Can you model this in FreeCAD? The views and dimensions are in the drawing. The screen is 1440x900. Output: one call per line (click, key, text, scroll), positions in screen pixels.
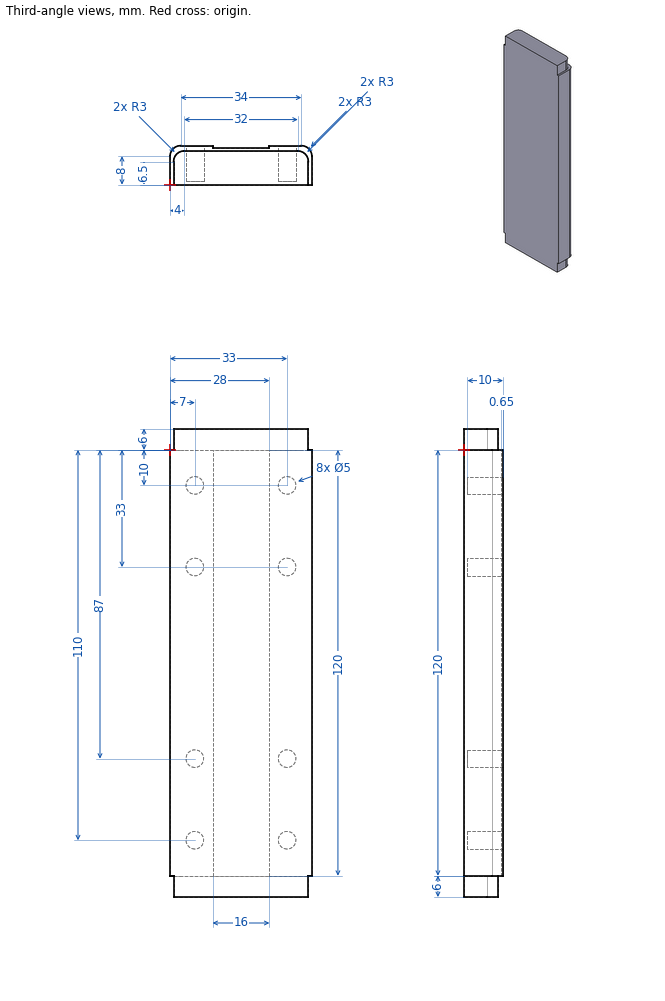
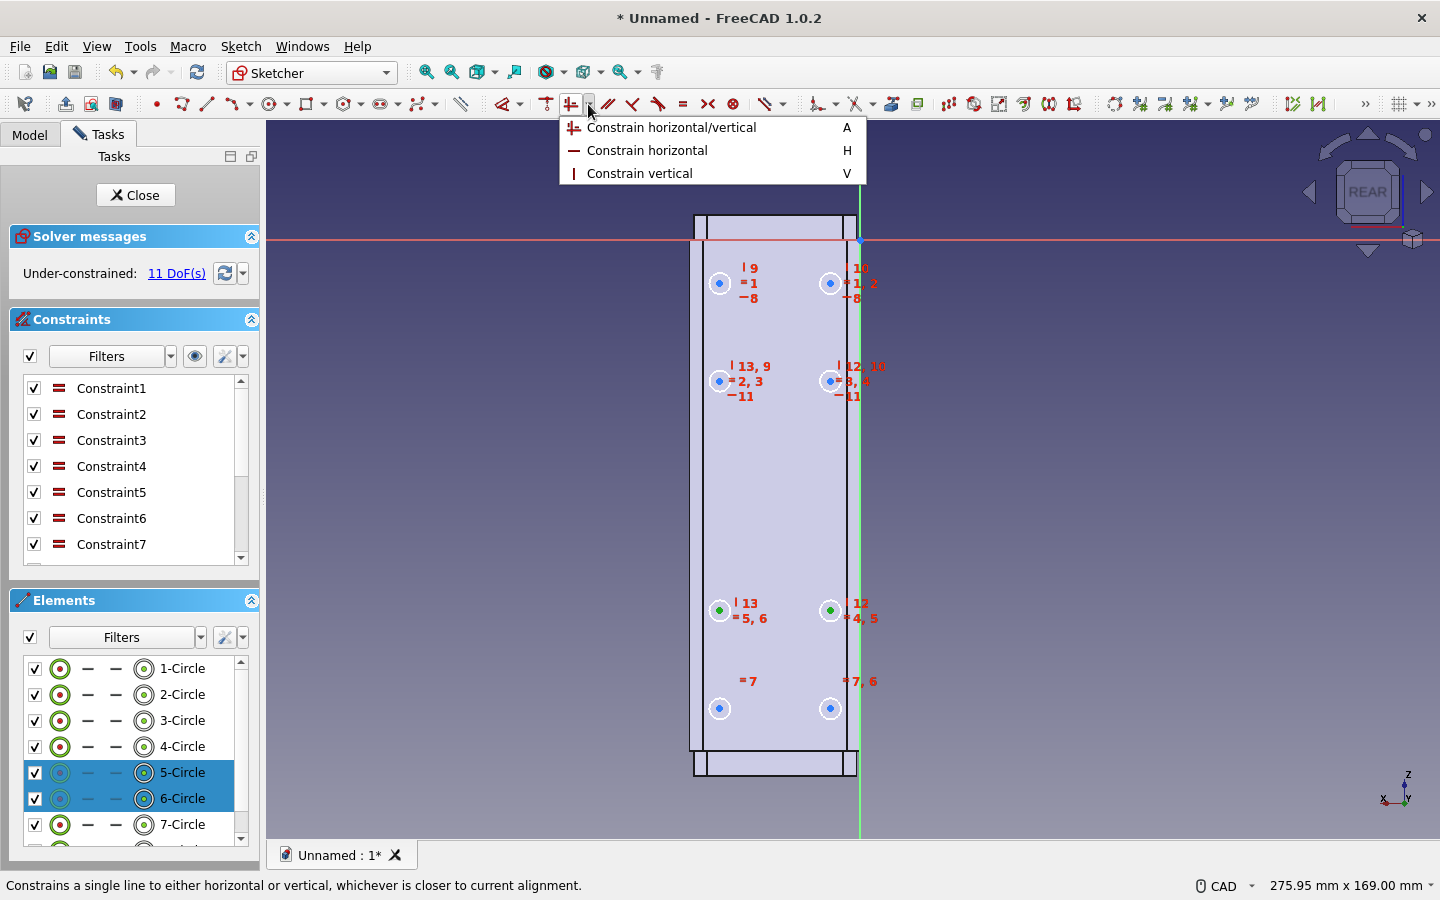
click(713, 150)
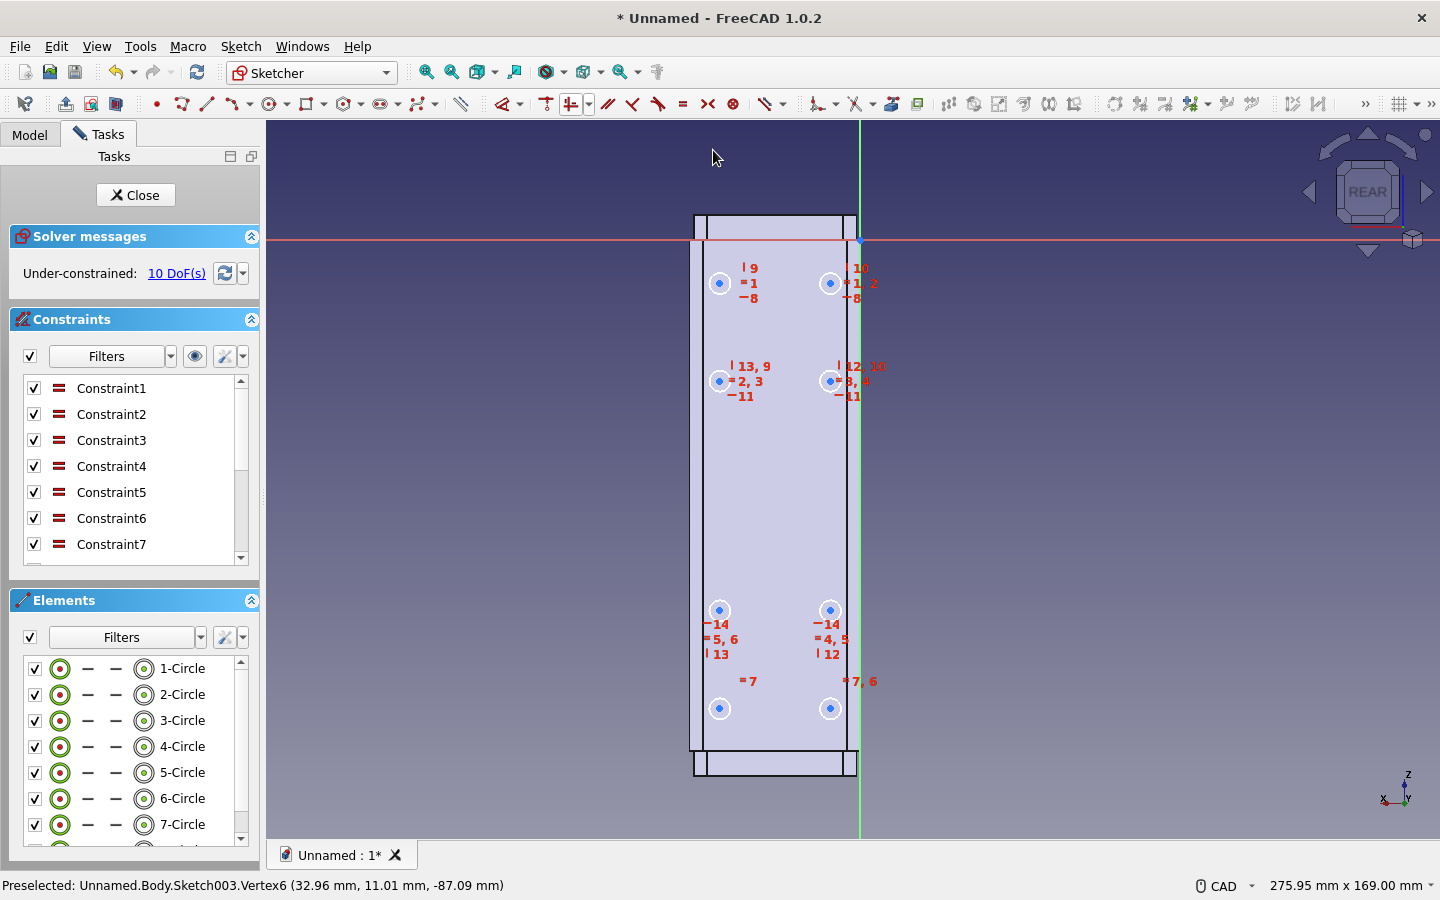
click(831, 611)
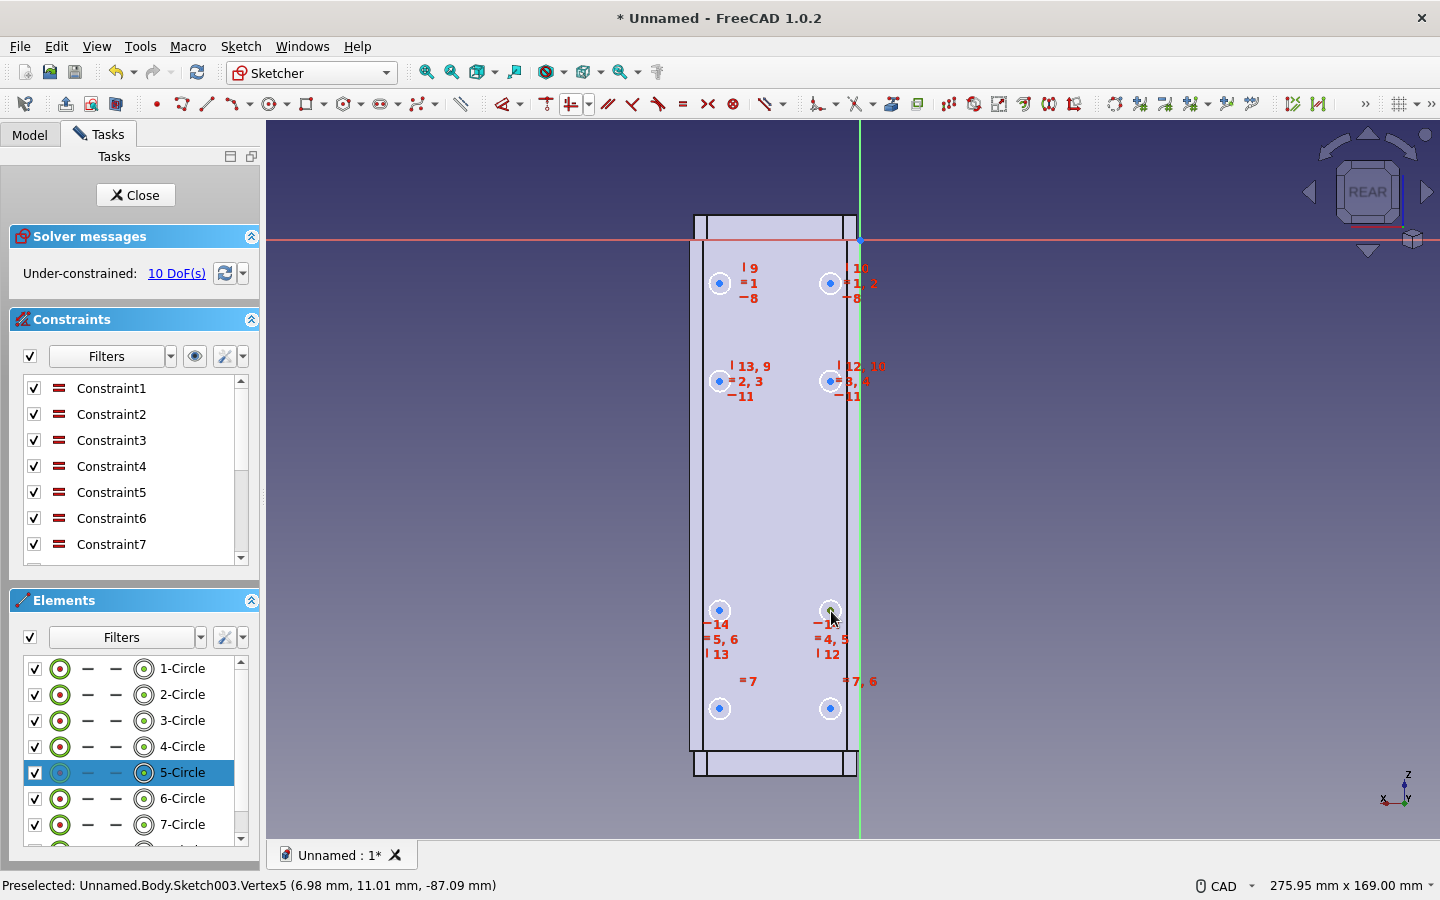
click(830, 709)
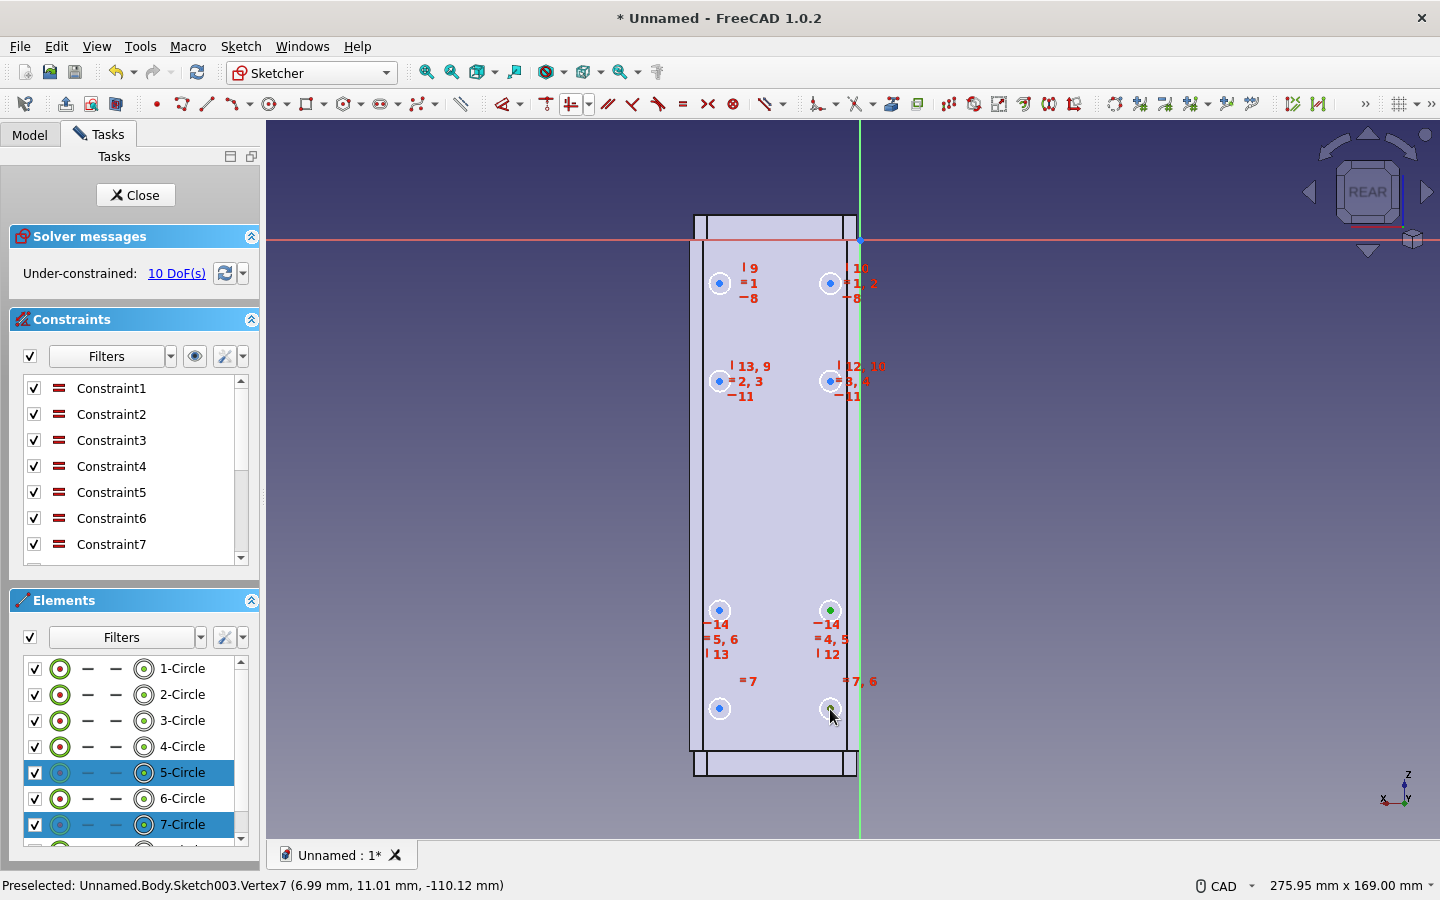
key(v)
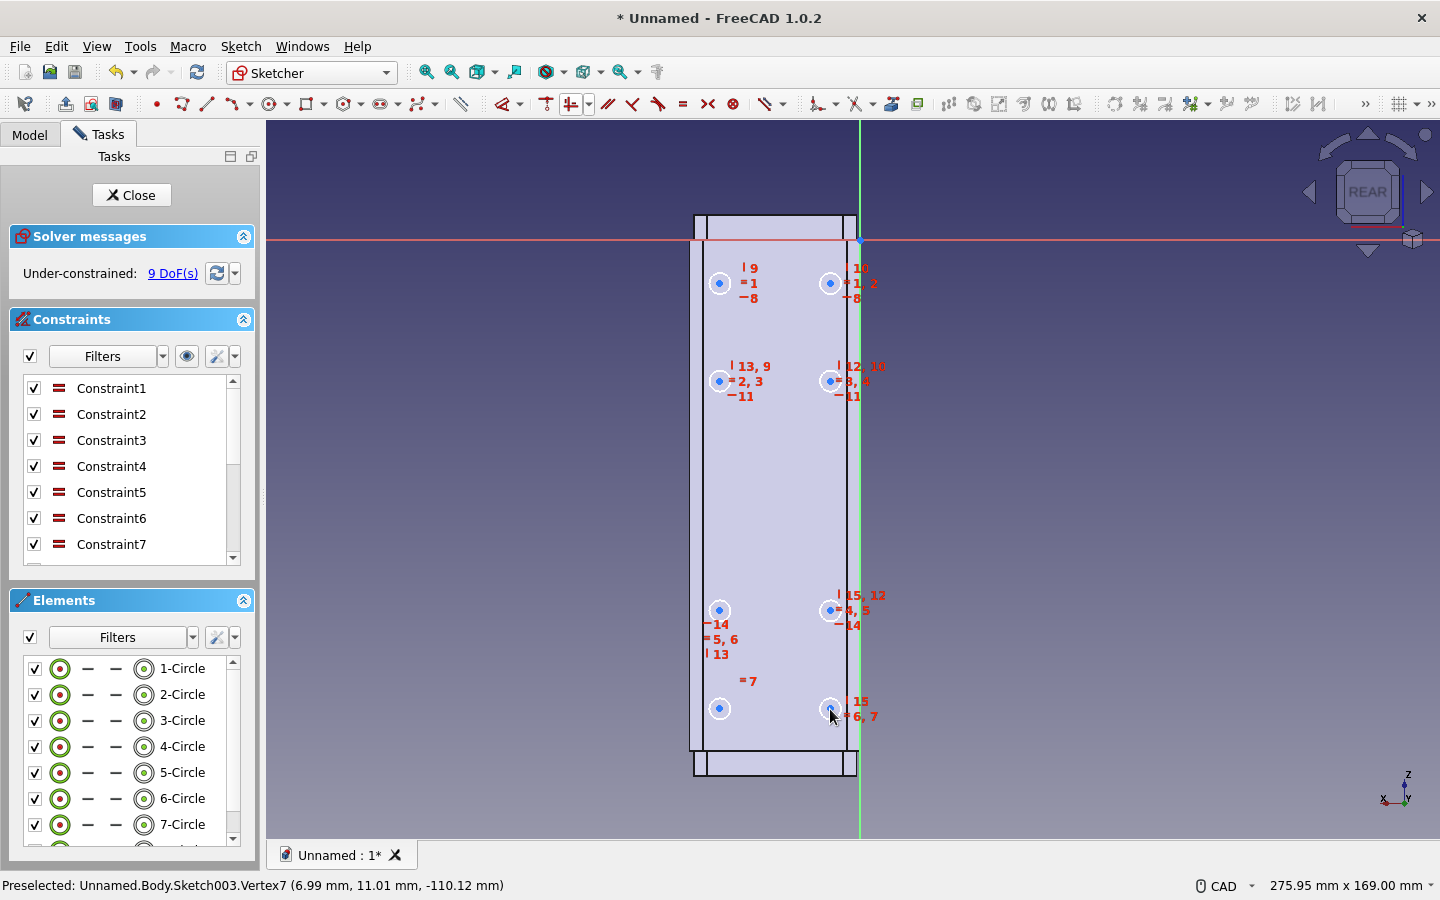
click(720, 611)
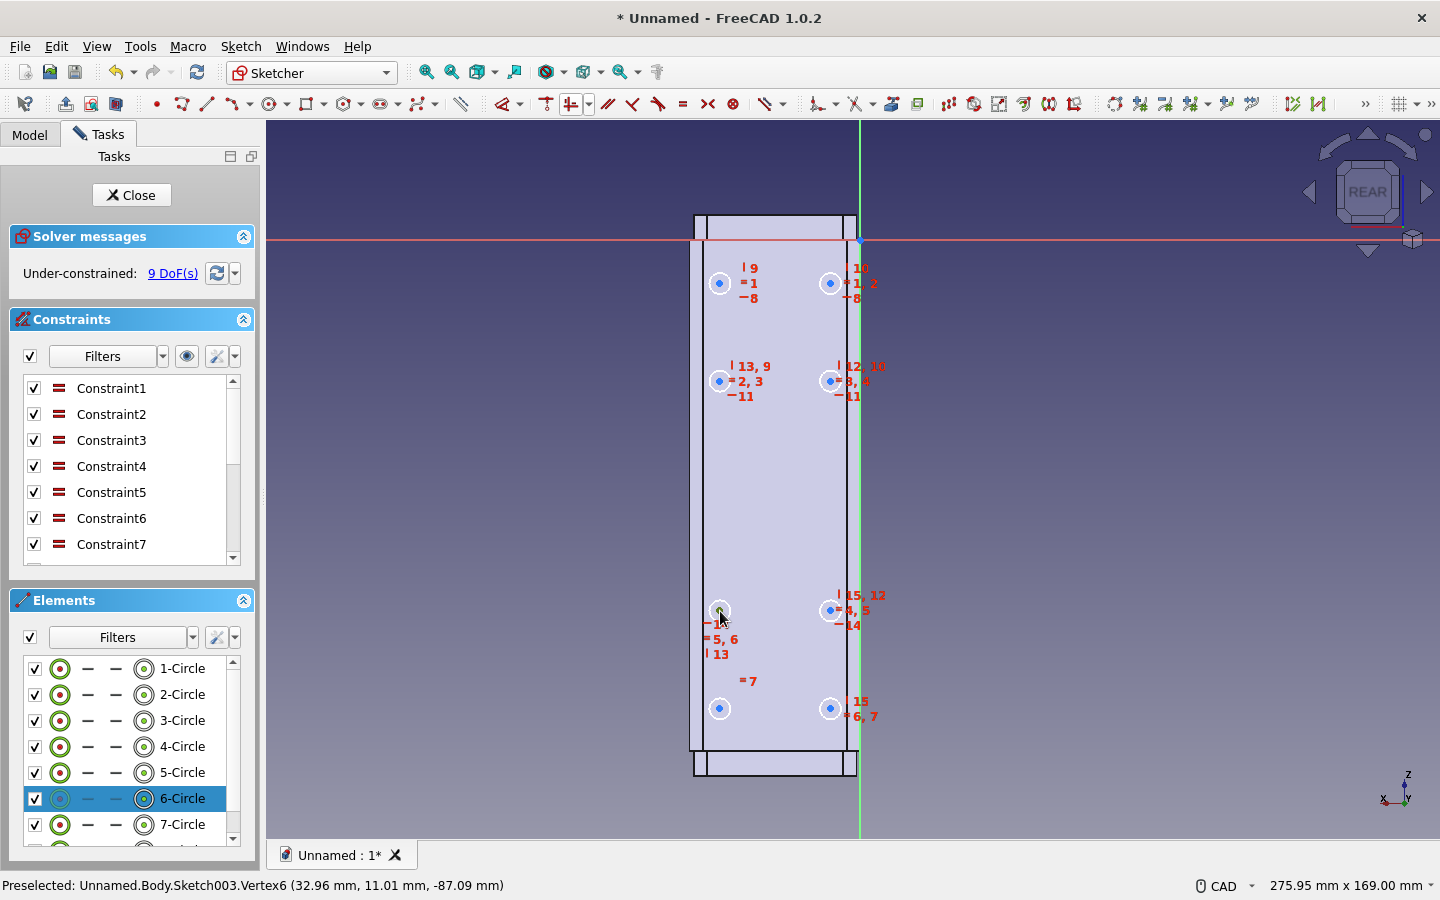
click(720, 709)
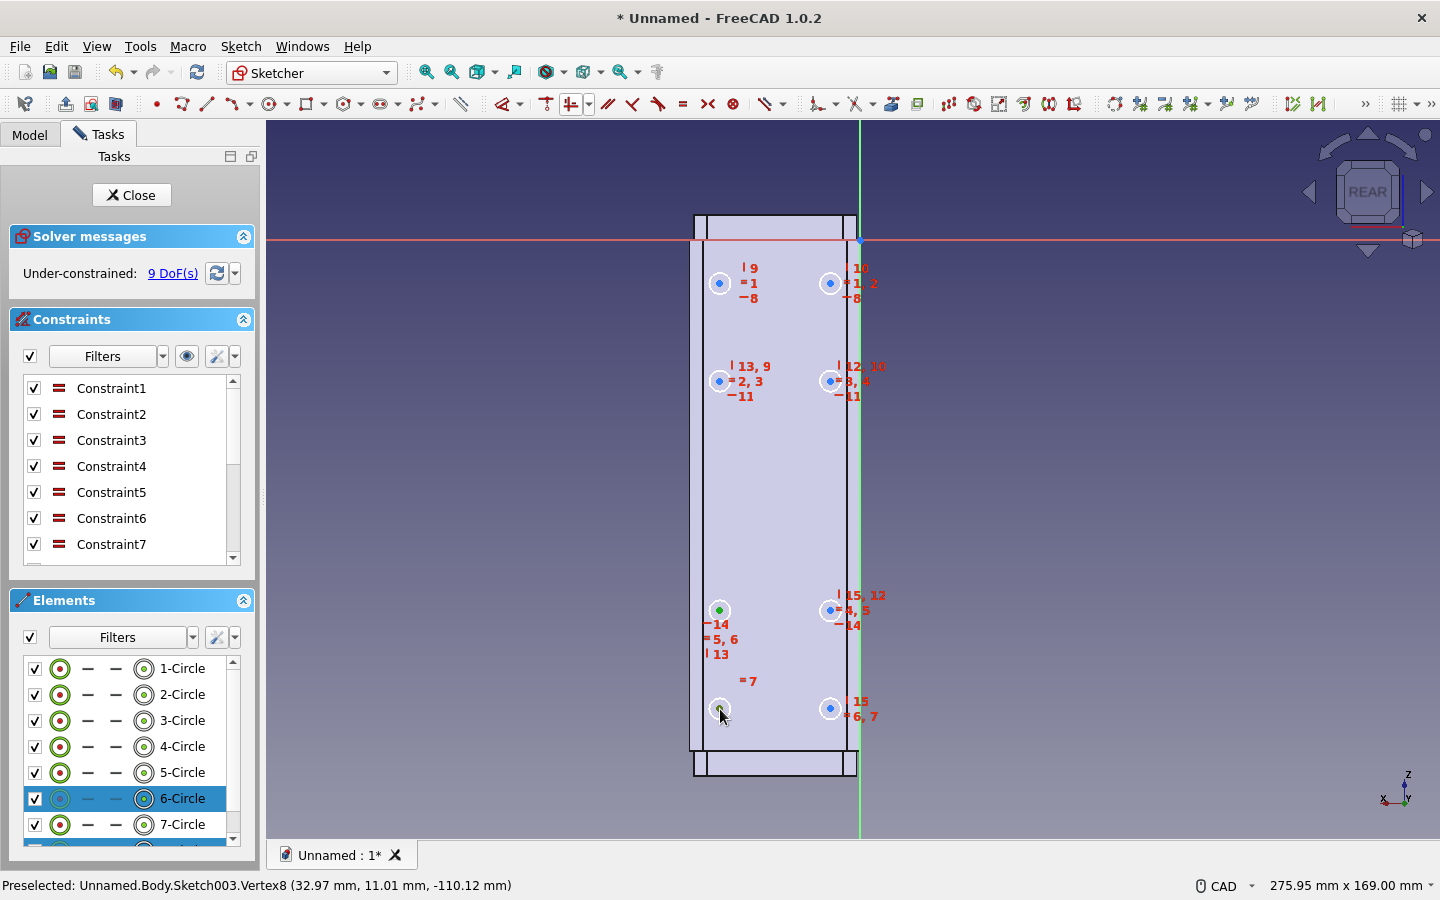
key(v)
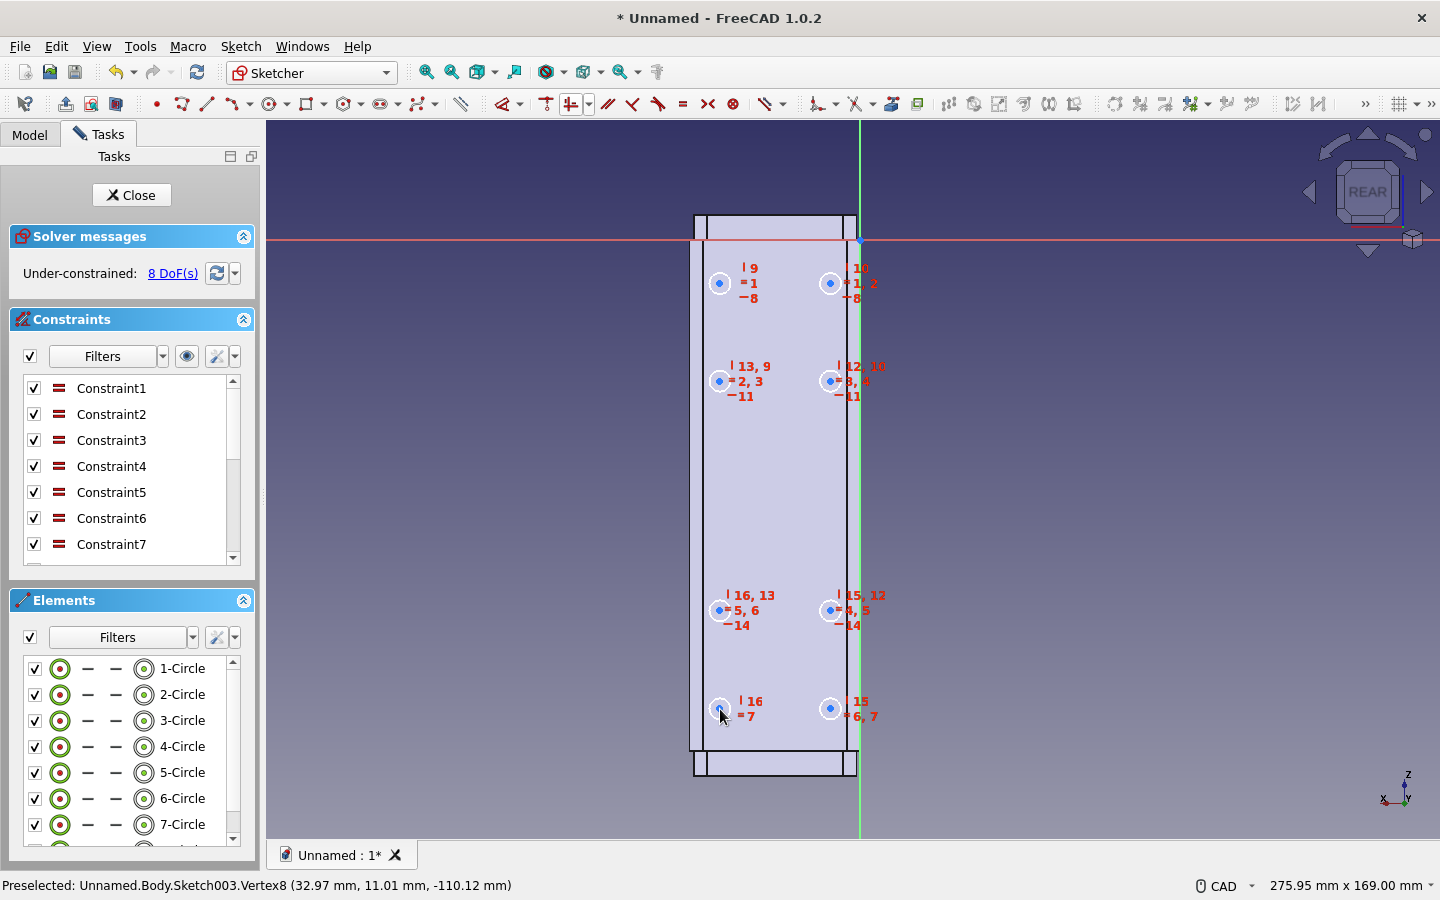
click(831, 709)